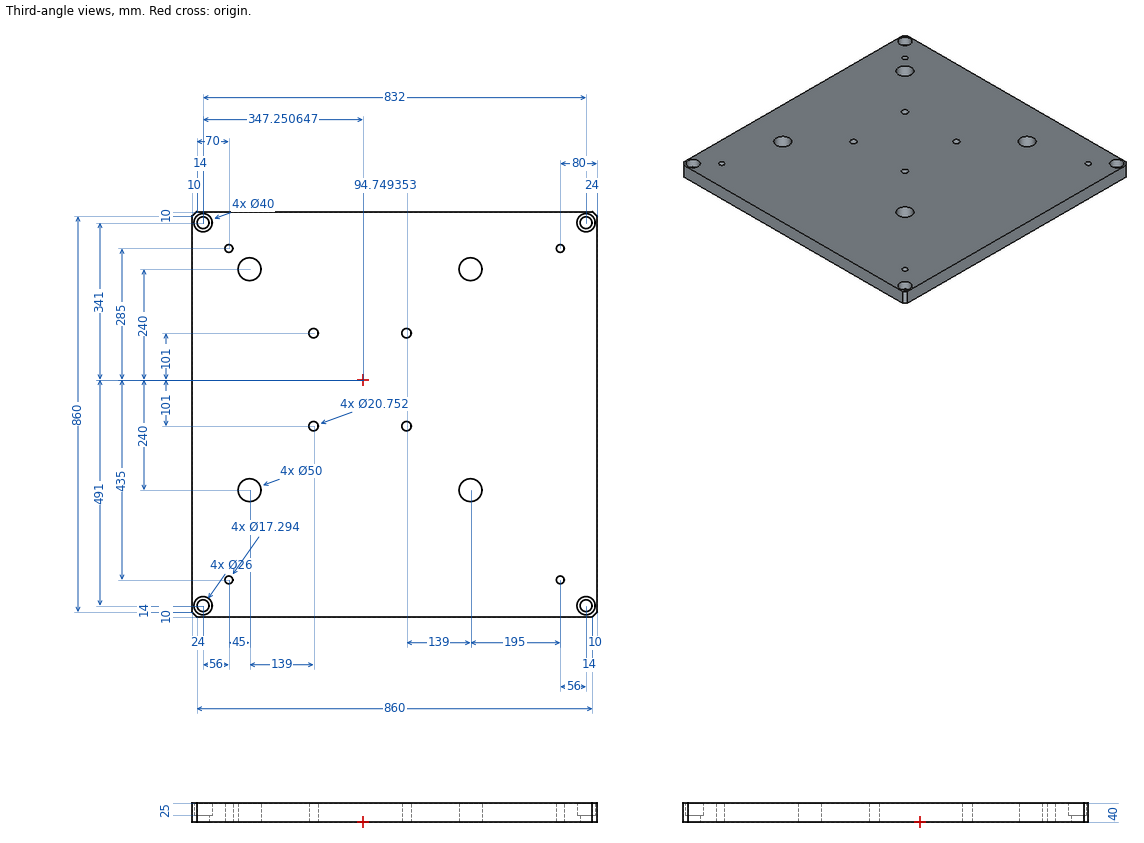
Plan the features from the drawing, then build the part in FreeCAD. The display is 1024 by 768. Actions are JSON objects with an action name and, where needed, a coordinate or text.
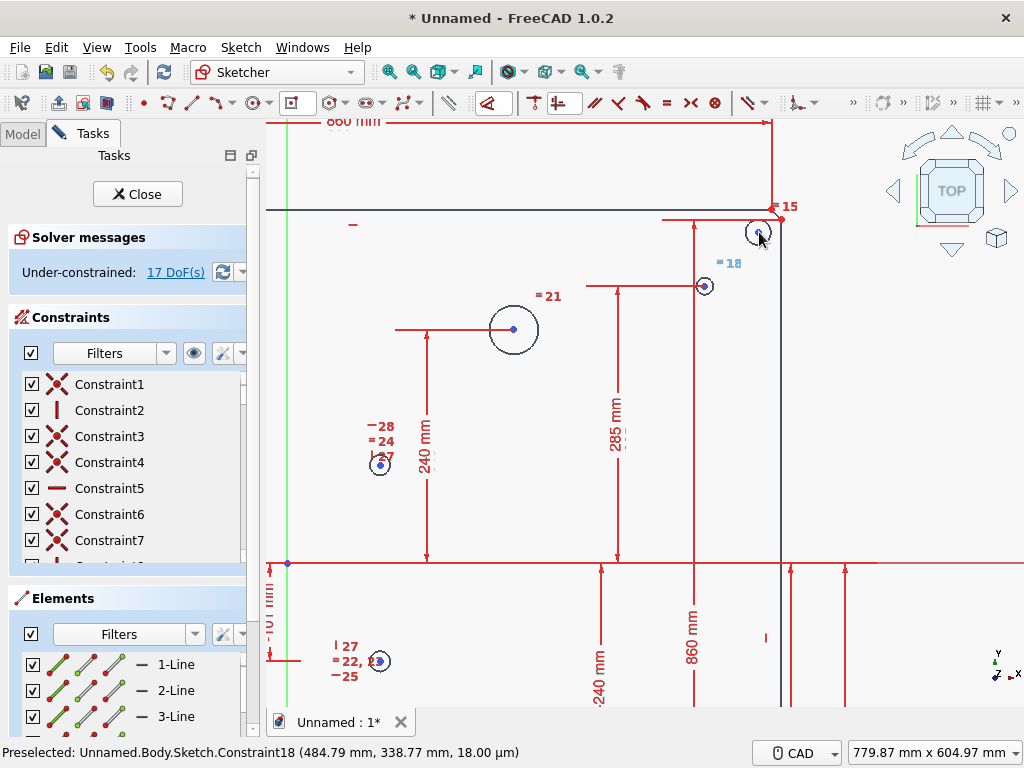
{"action": "left_click", "coordinate": [758, 232]}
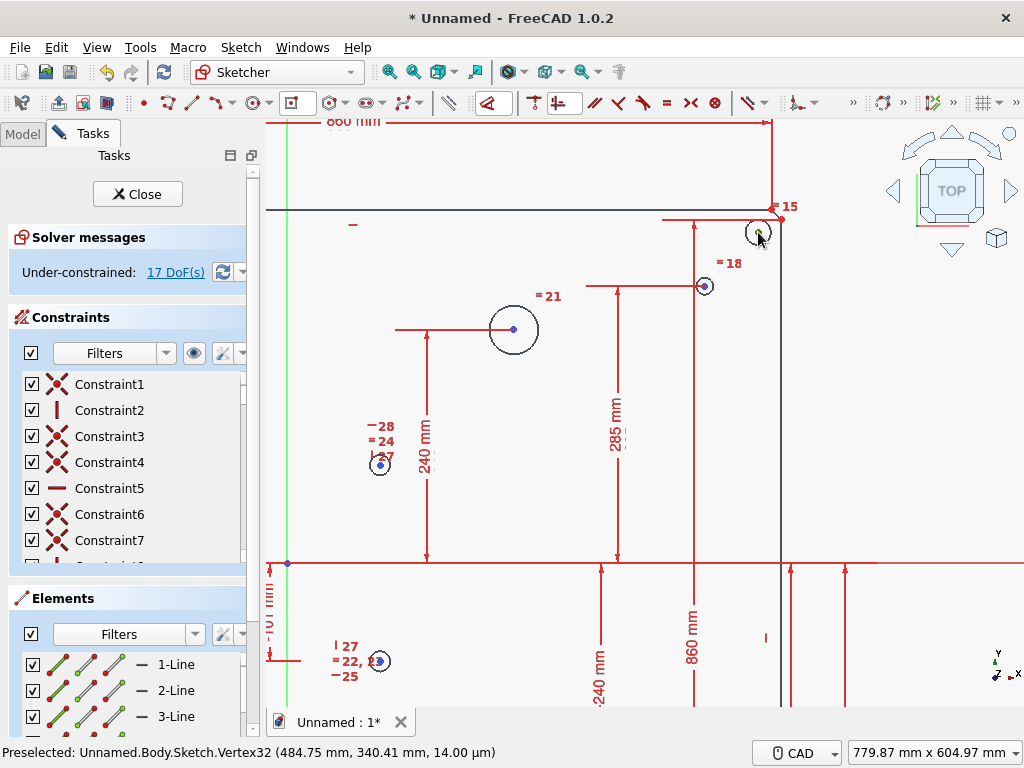
{"action": "key", "text": "i"}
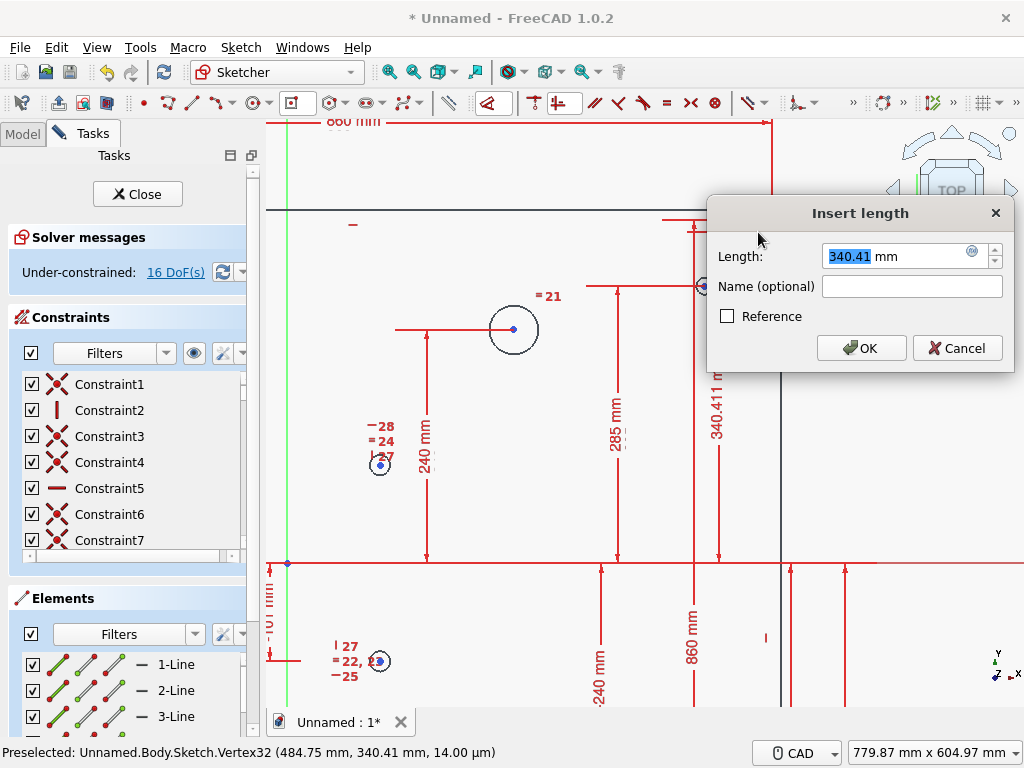
{"action": "type", "text": "341"}
{"action": "key", "text": "Return"}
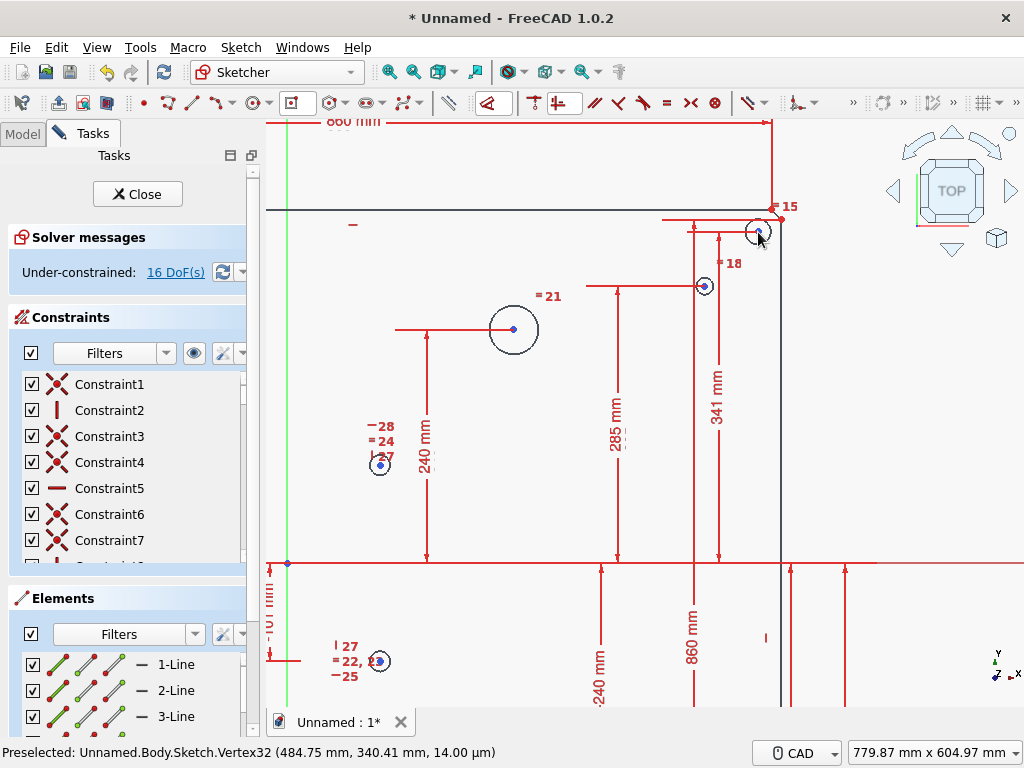
{"action": "scroll", "coordinate": [758, 231], "scroll_direction": "down", "scroll_amount": 4}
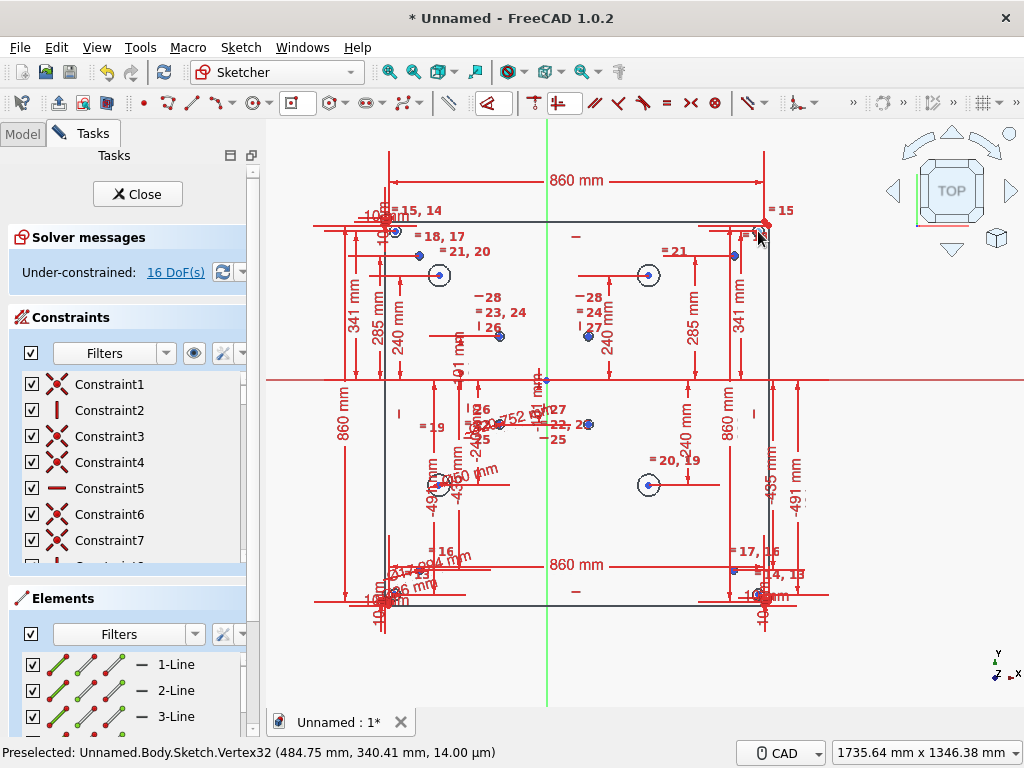
{"action": "scroll", "coordinate": [385, 602], "scroll_direction": "up", "scroll_amount": 7}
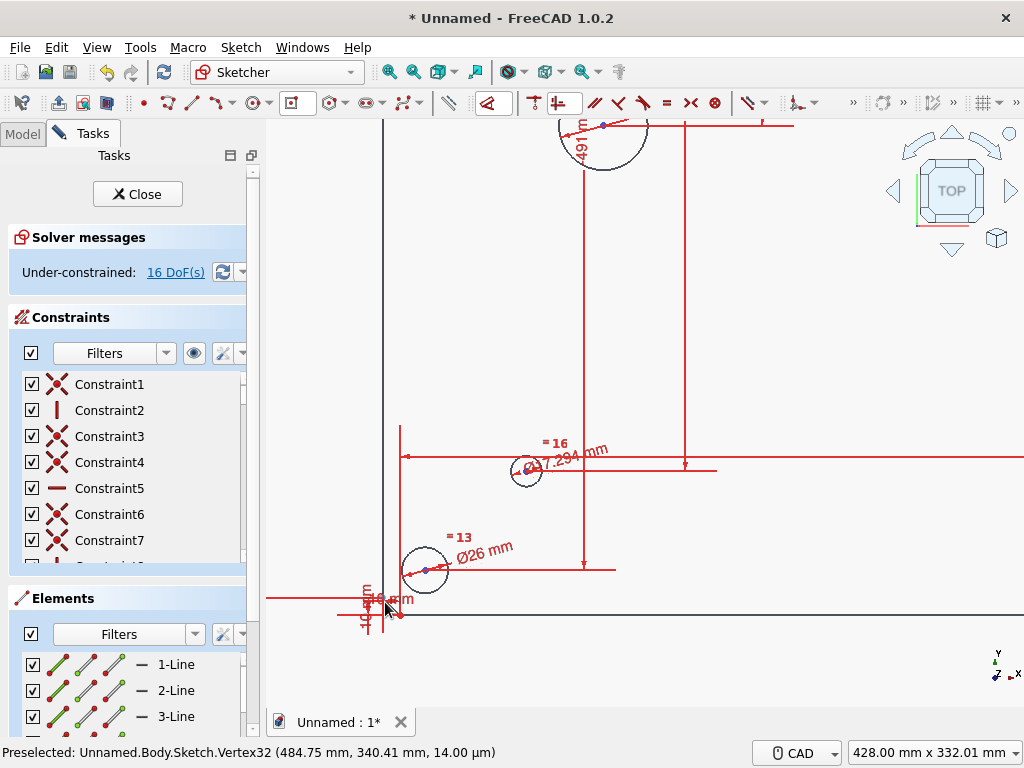
{"action": "left_click", "coordinate": [383, 598]}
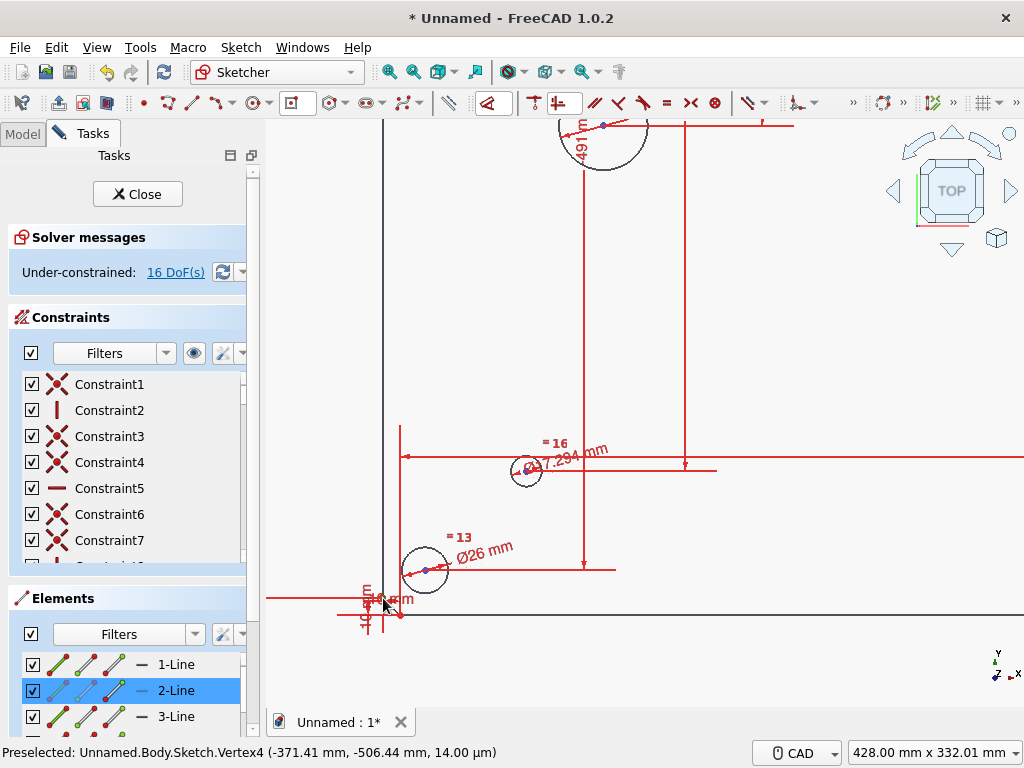
{"action": "left_click", "coordinate": [425, 570]}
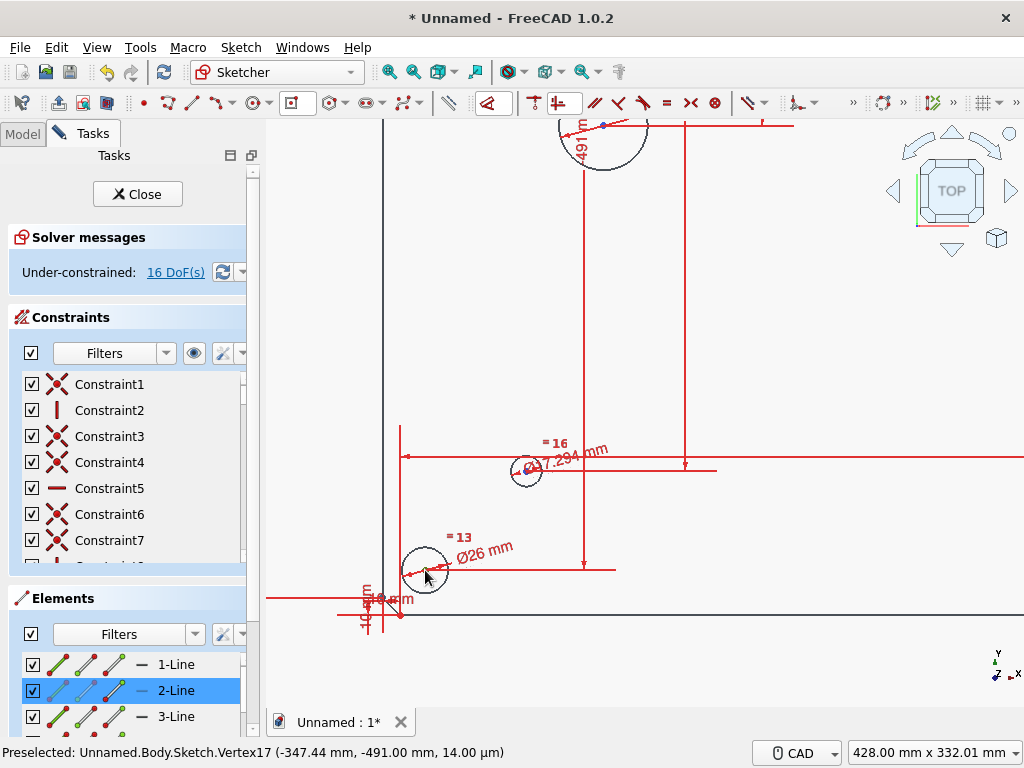
{"action": "key", "text": "l"}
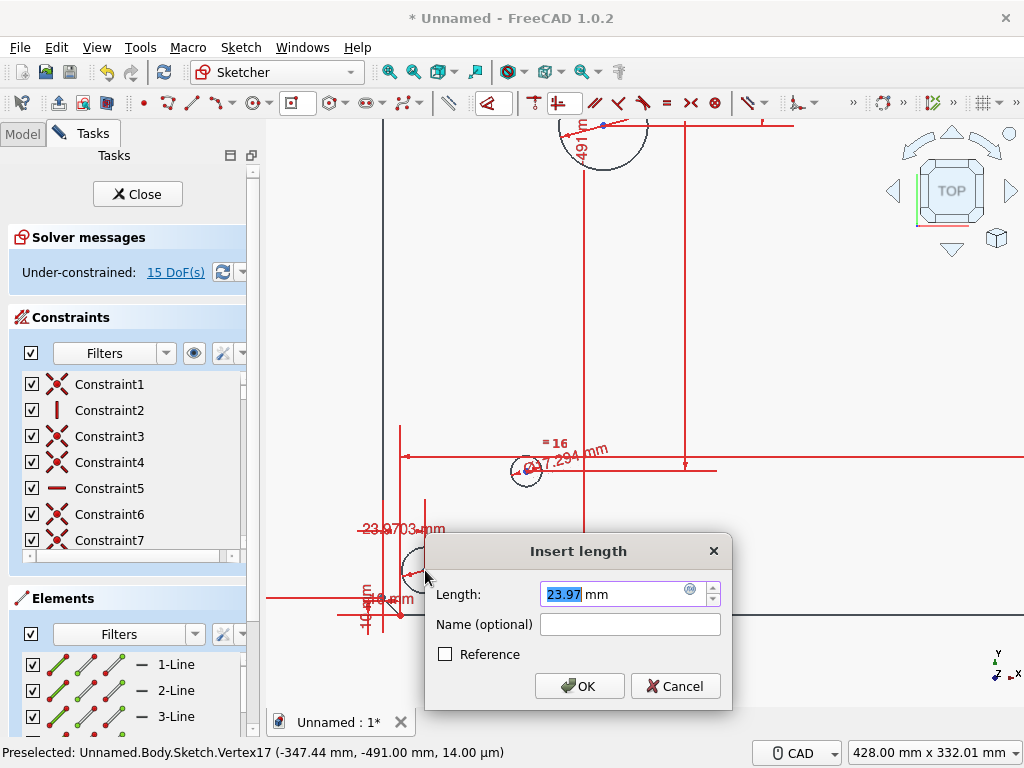
{"action": "type", "text": "24"}
{"action": "key", "text": "Return"}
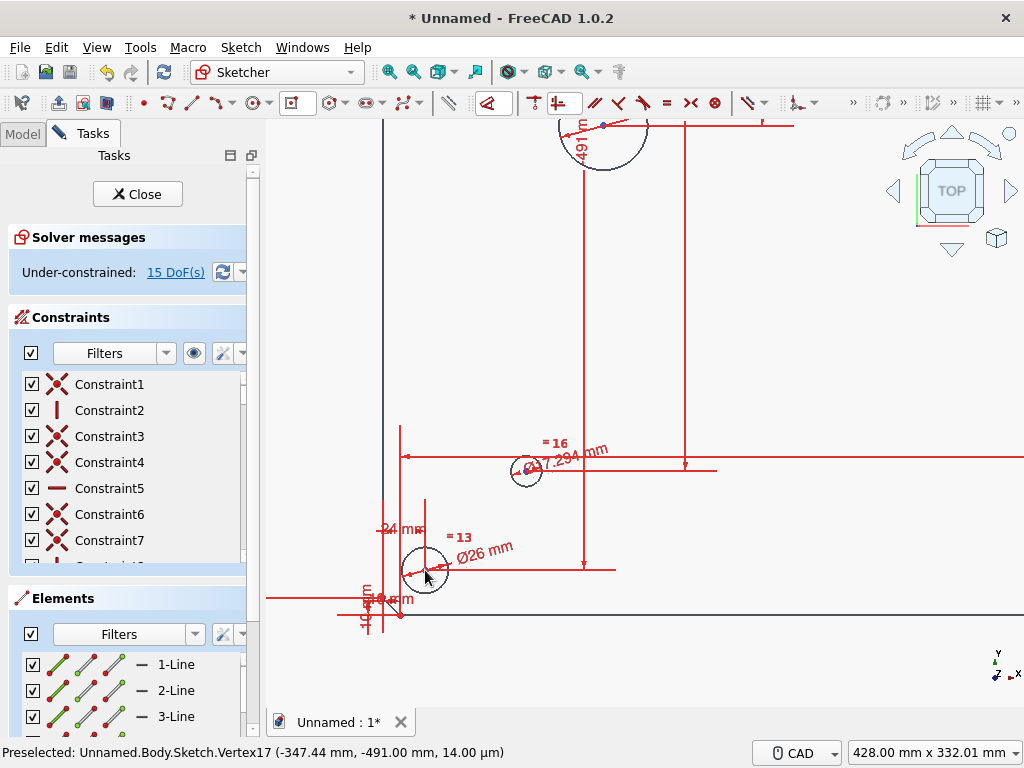
{"action": "scroll", "coordinate": [383, 598], "scroll_direction": "up", "scroll_amount": 3}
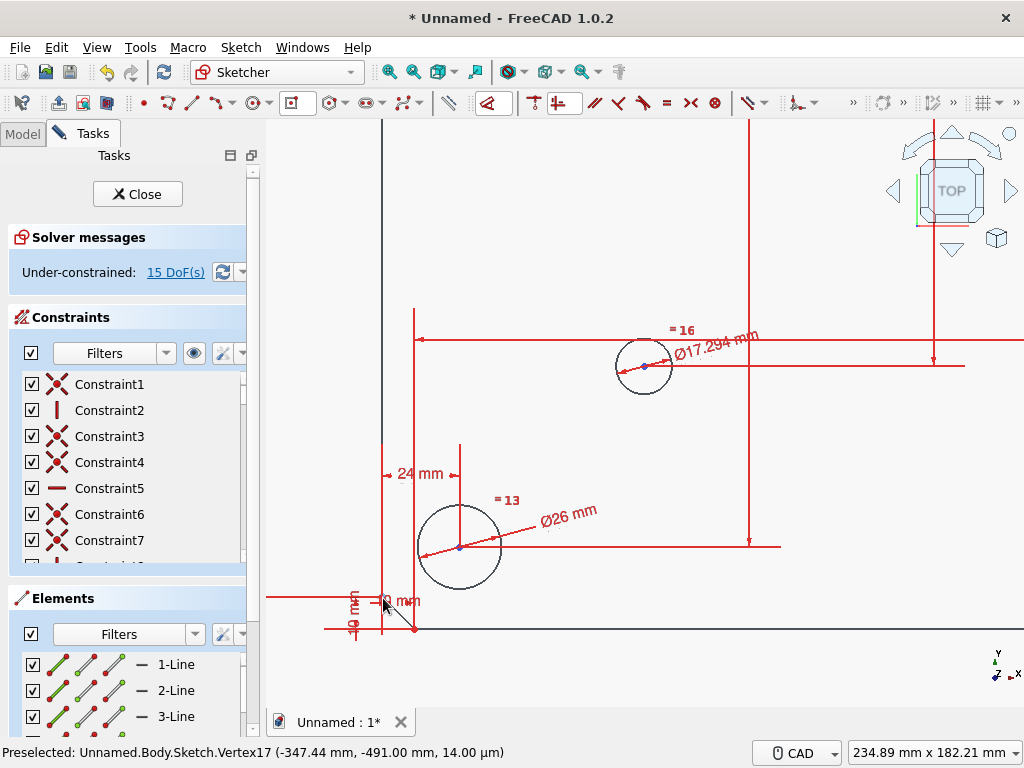
{"action": "left_click", "coordinate": [382, 597]}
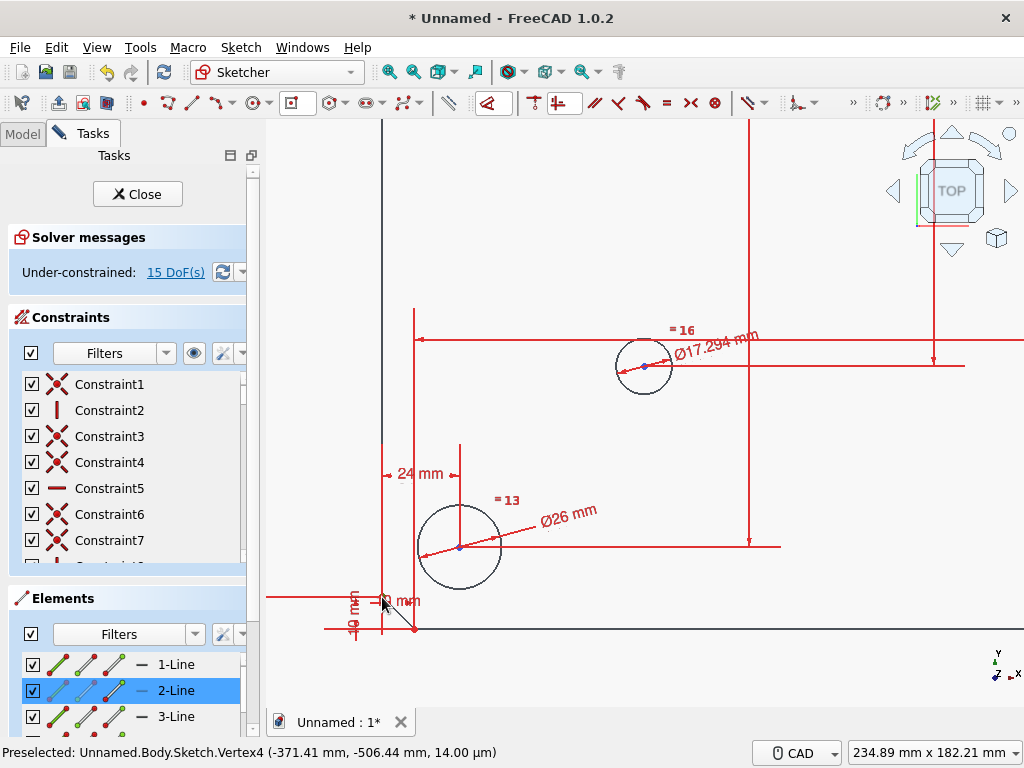
{"action": "left_click", "coordinate": [460, 547]}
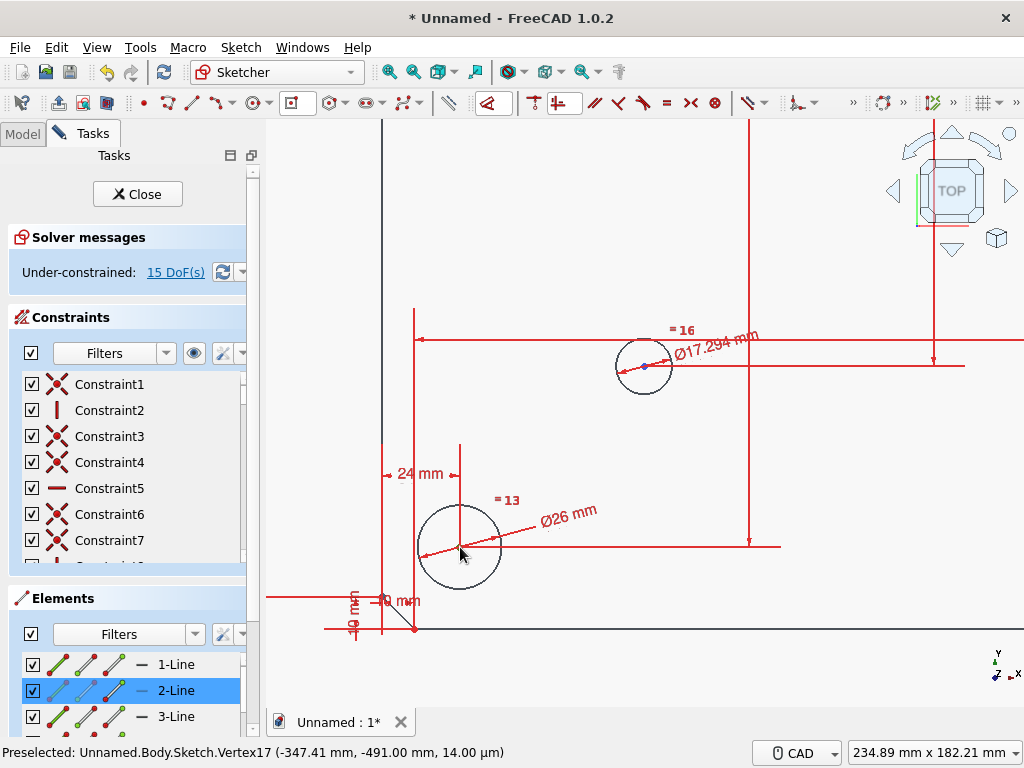
{"action": "key", "text": "i"}